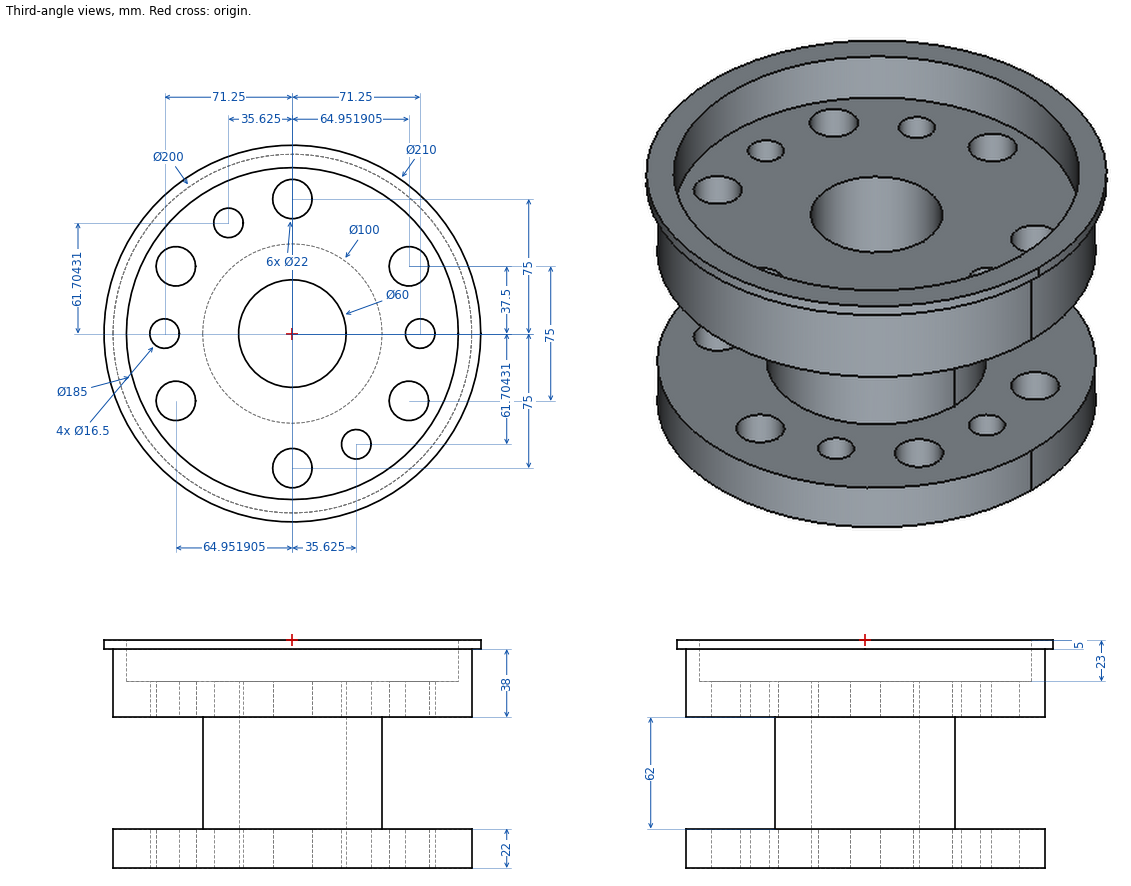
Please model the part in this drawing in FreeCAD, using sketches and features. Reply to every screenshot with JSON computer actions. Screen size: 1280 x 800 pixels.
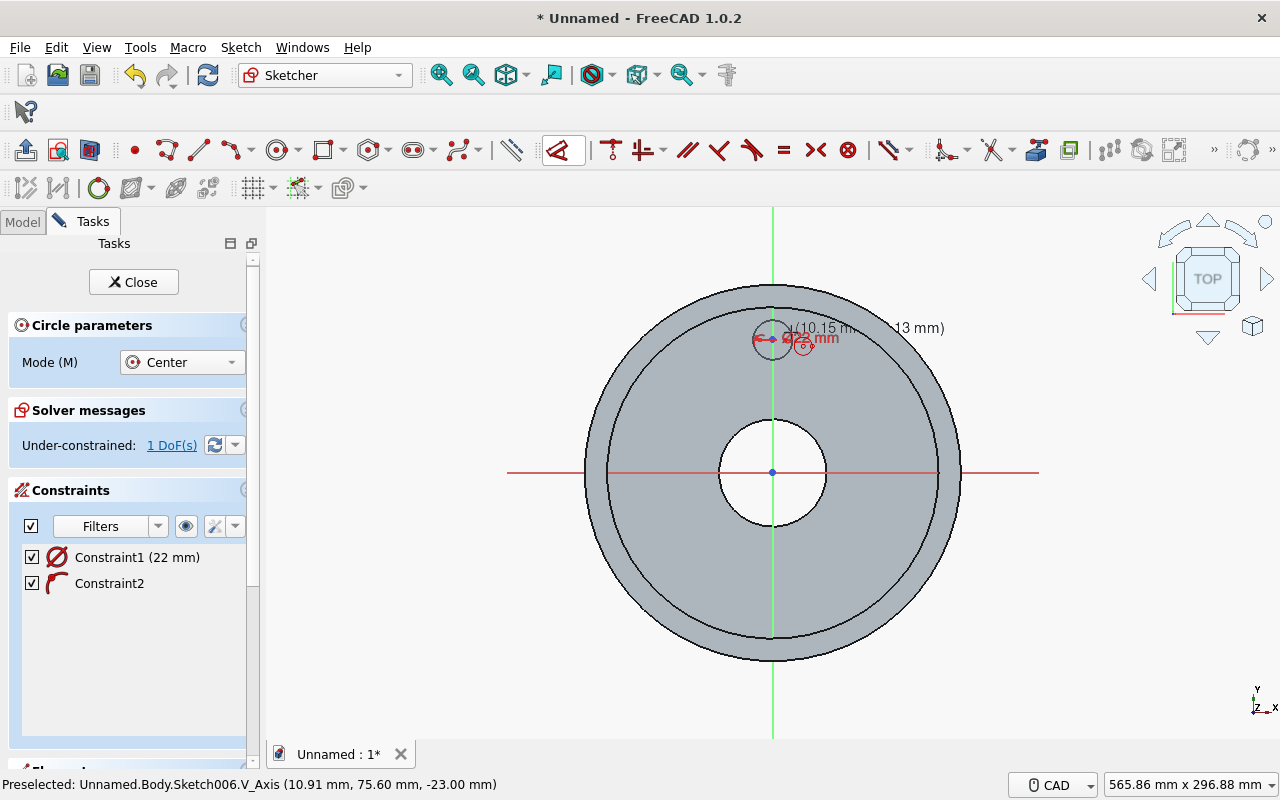
{"action": "left_click", "coordinate": [889, 406]}
{"action": "mouse_move", "coordinate": [903, 392]}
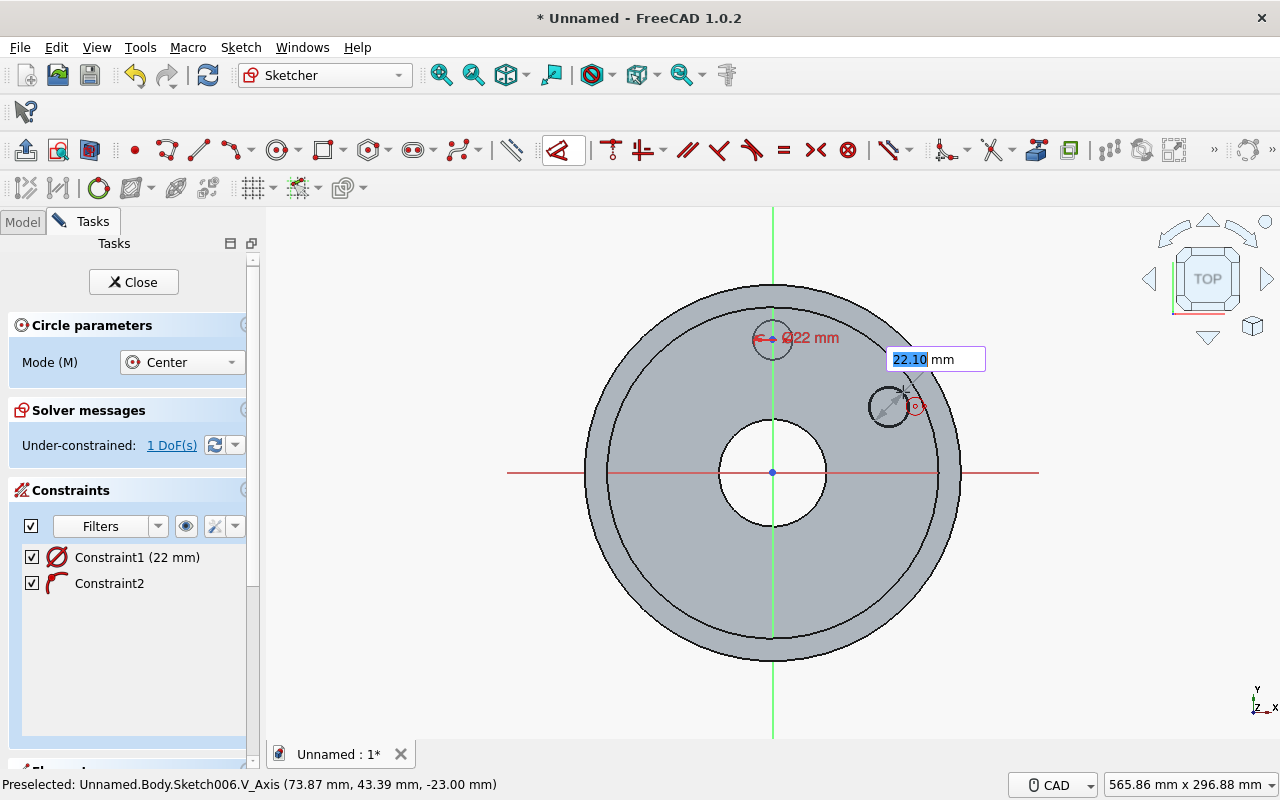
{"action": "type", "text": "22"}
{"action": "key", "text": "Return"}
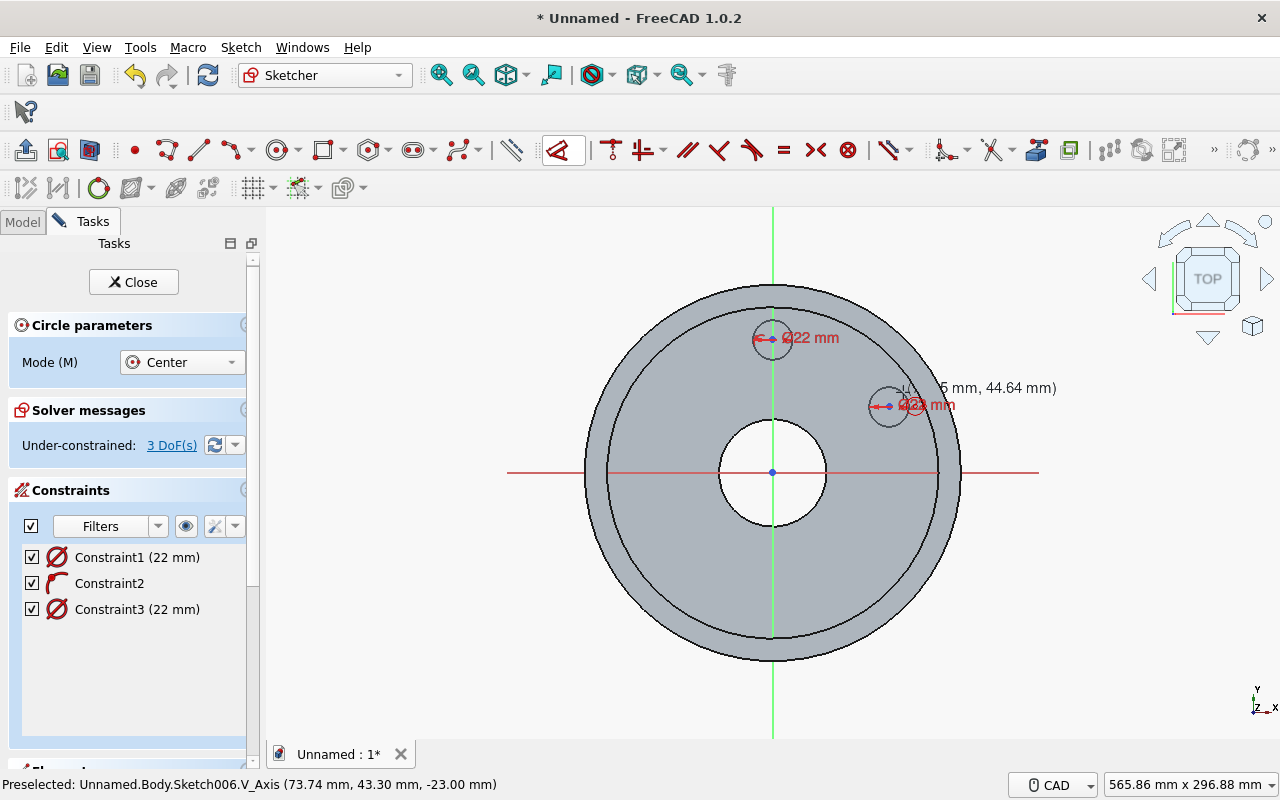
{"action": "left_click", "coordinate": [889, 540]}
{"action": "mouse_move", "coordinate": [903, 526]}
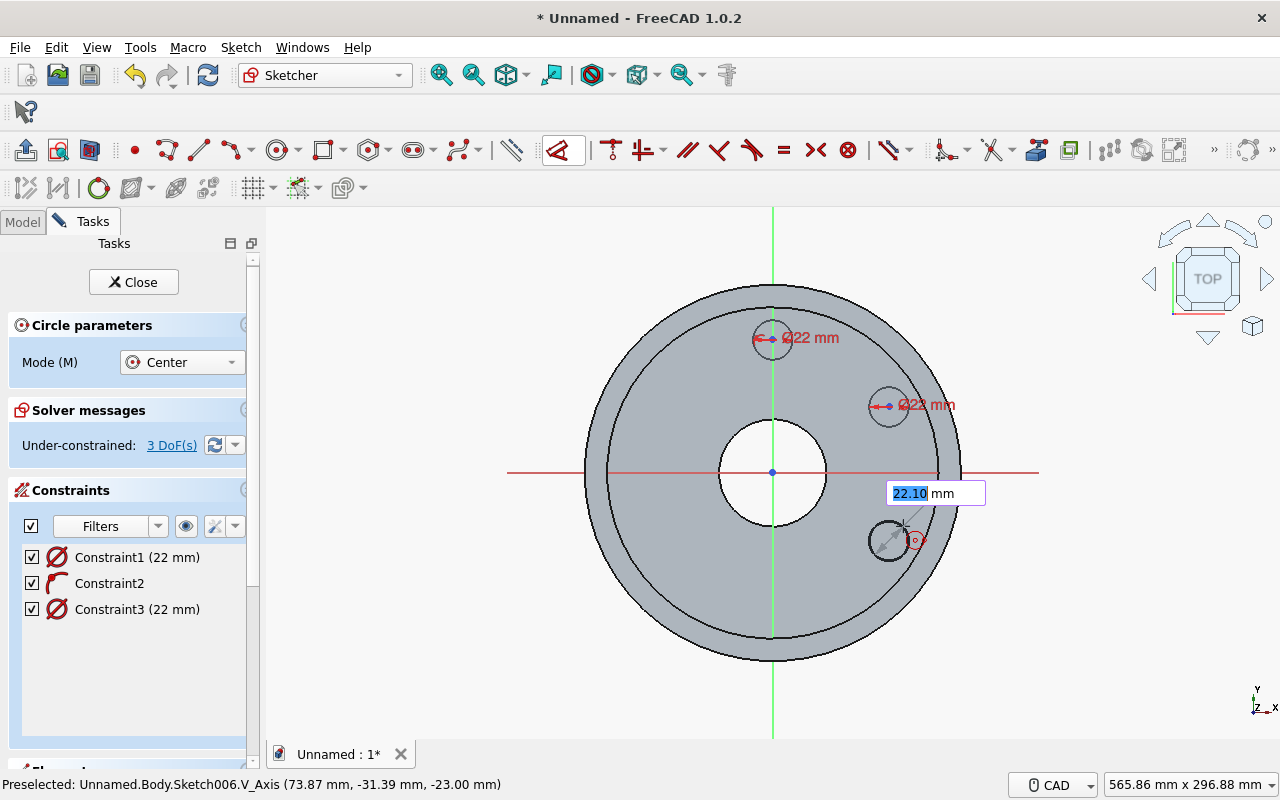
{"action": "type", "text": "22"}
{"action": "key", "text": "Return"}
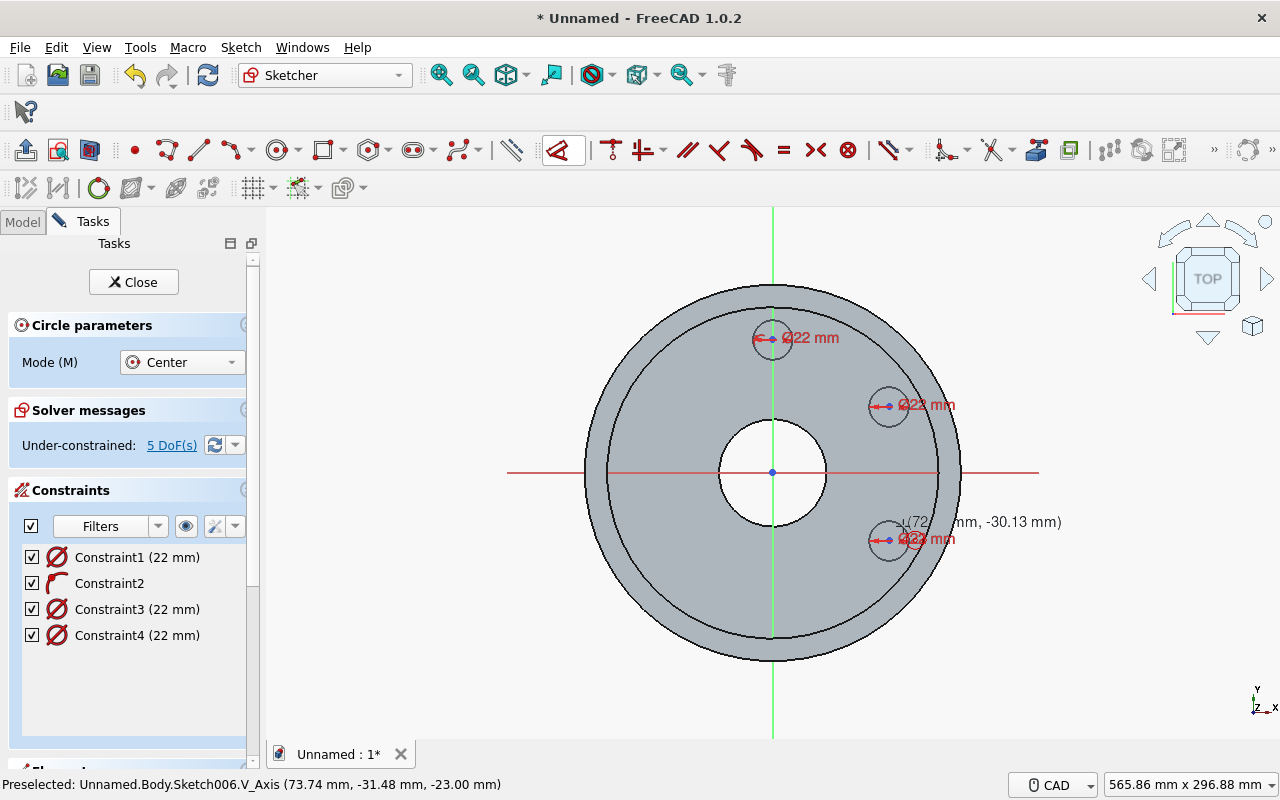
{"action": "left_click", "coordinate": [773, 607]}
{"action": "mouse_move", "coordinate": [791, 601]}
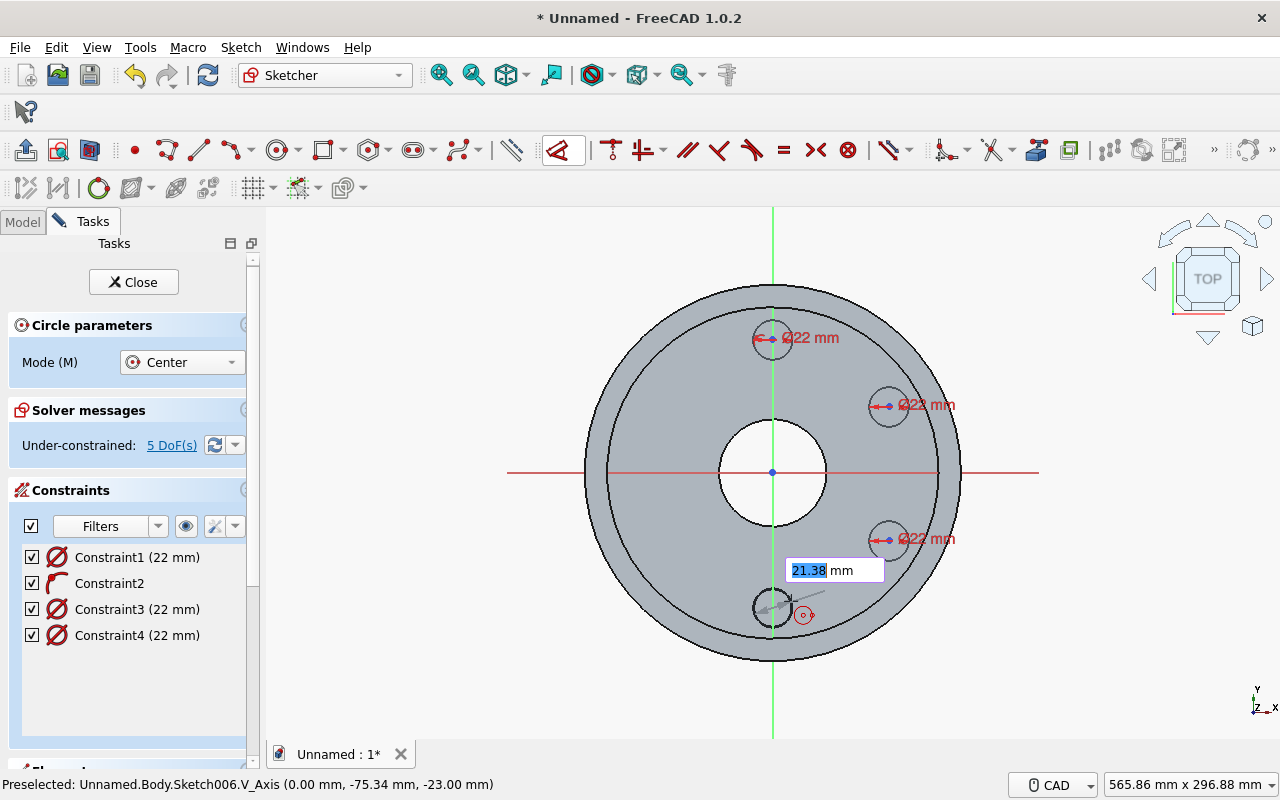
{"action": "type", "text": "22"}
{"action": "key", "text": "Return"}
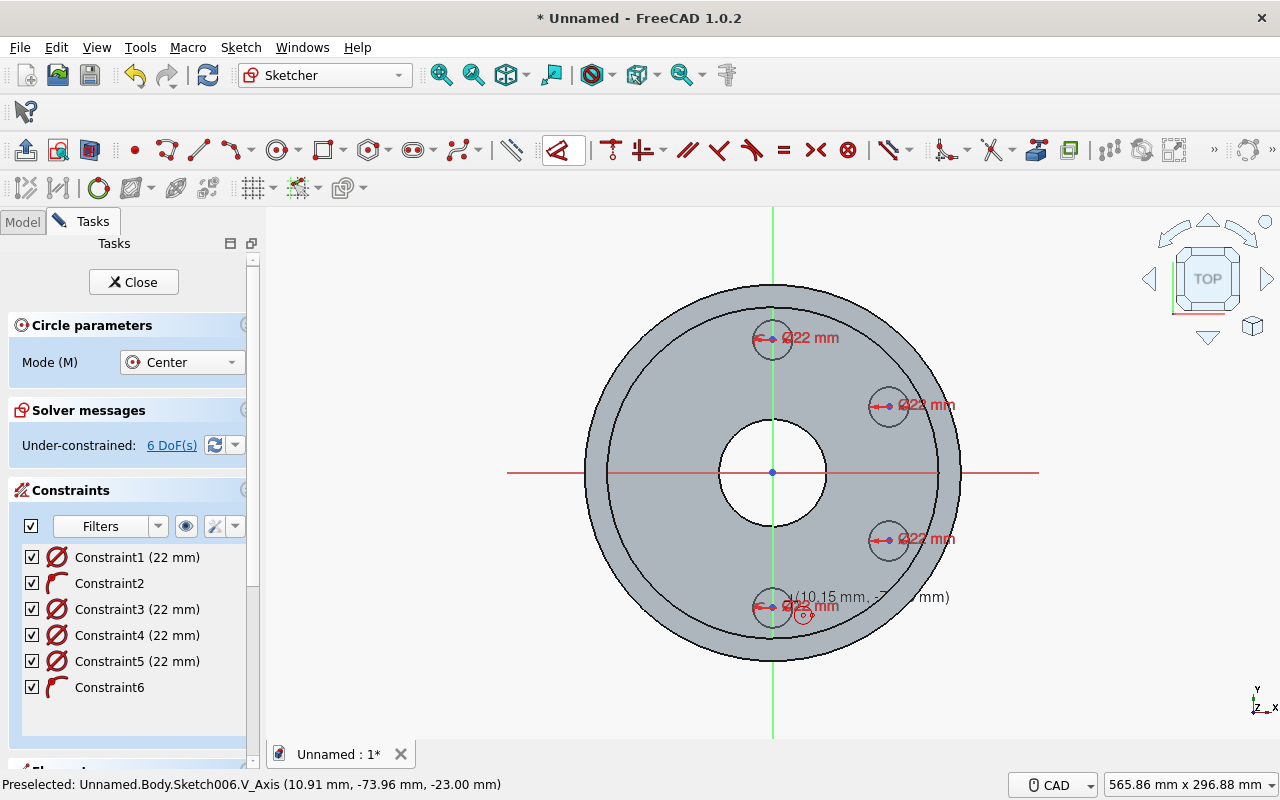
{"action": "left_click", "coordinate": [656, 540]}
{"action": "mouse_move", "coordinate": [670, 526]}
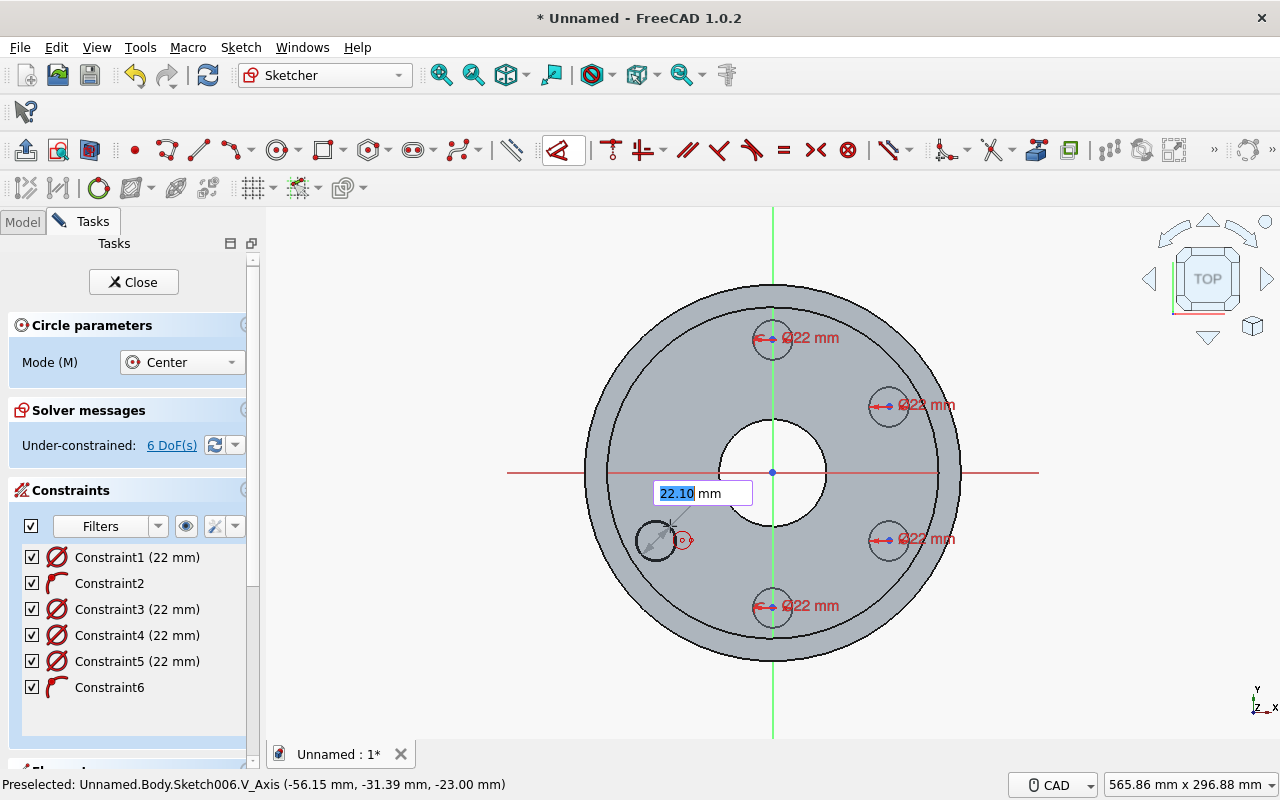
{"action": "type", "text": "22"}
{"action": "key", "text": "Return"}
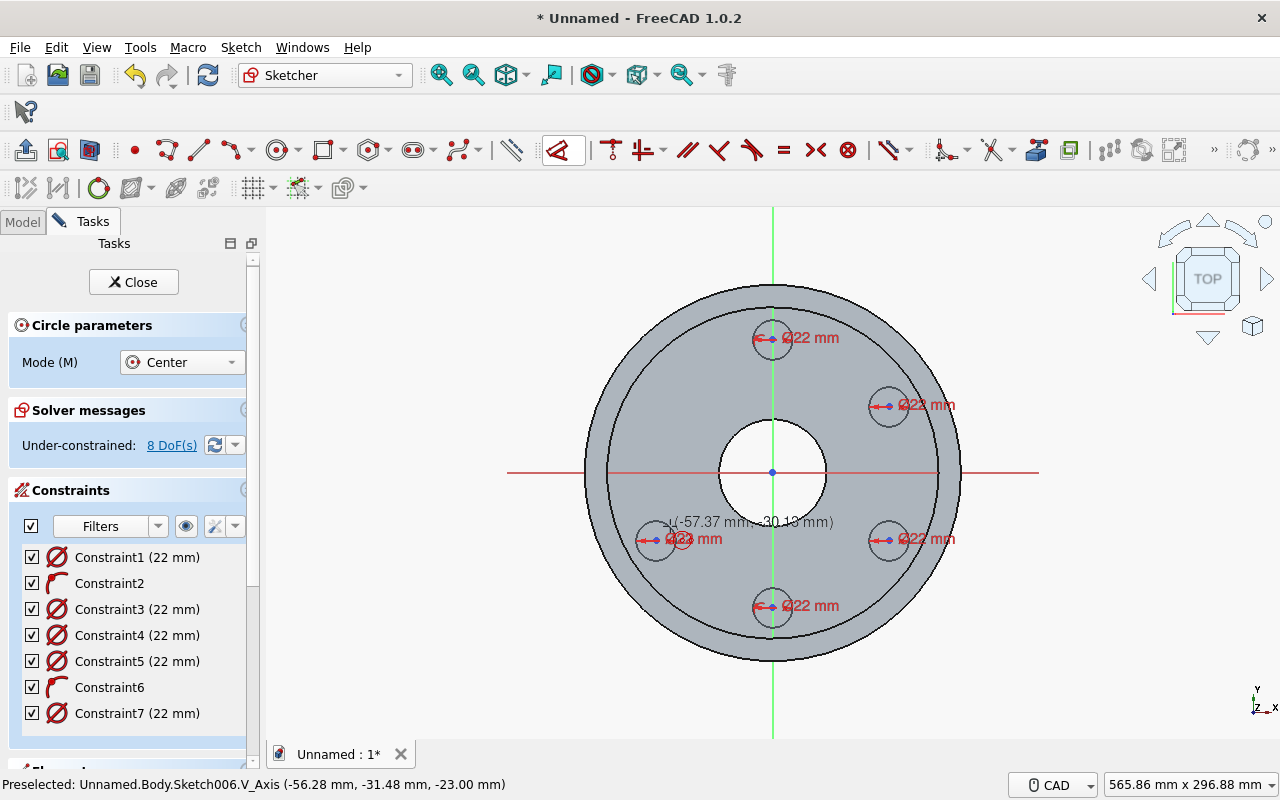
{"action": "left_click", "coordinate": [656, 406]}
{"action": "mouse_move", "coordinate": [670, 392]}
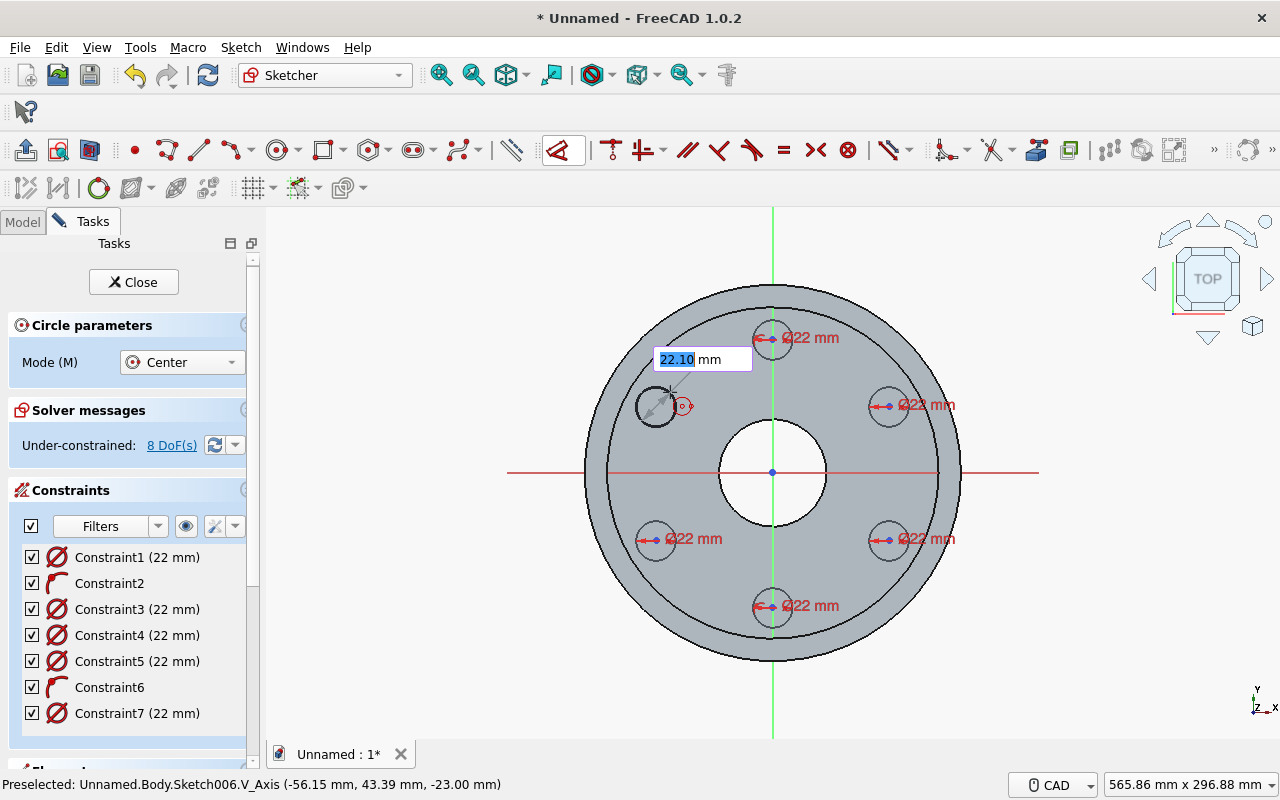
{"action": "type", "text": "22"}
{"action": "key", "text": "Return"}